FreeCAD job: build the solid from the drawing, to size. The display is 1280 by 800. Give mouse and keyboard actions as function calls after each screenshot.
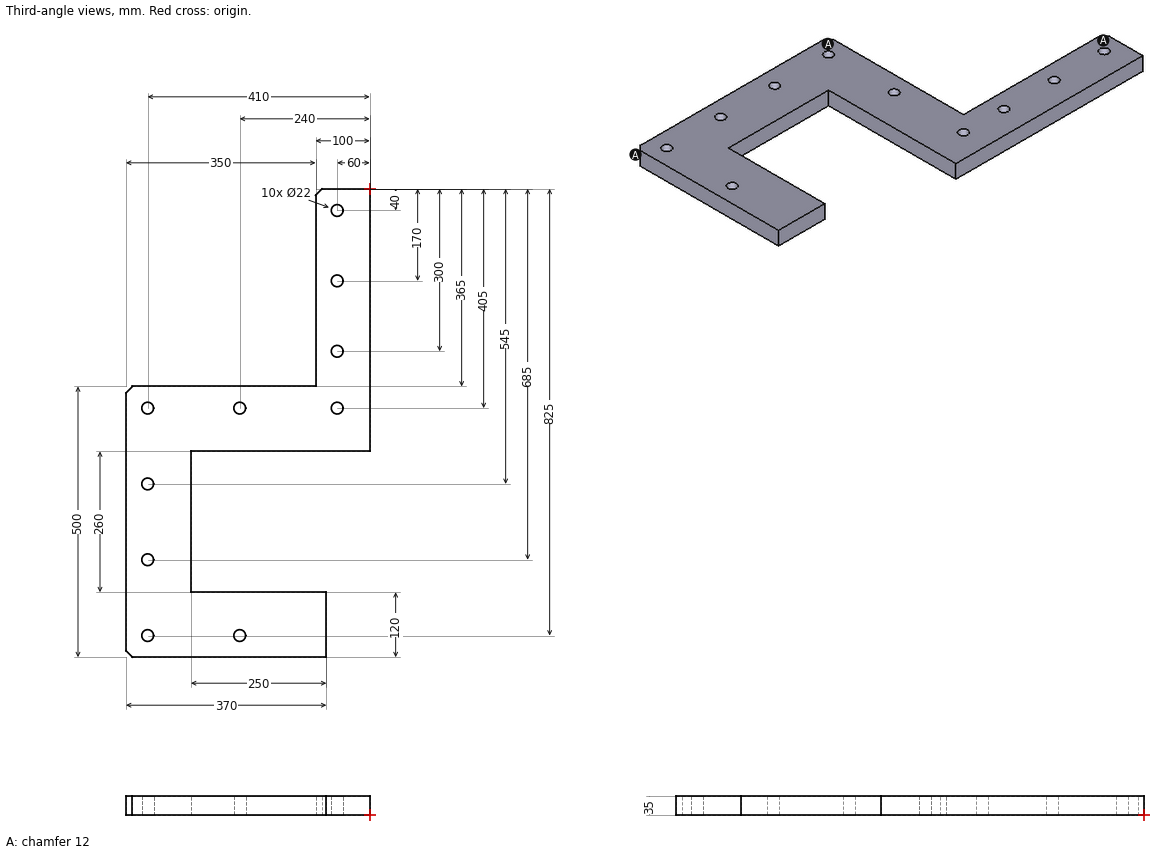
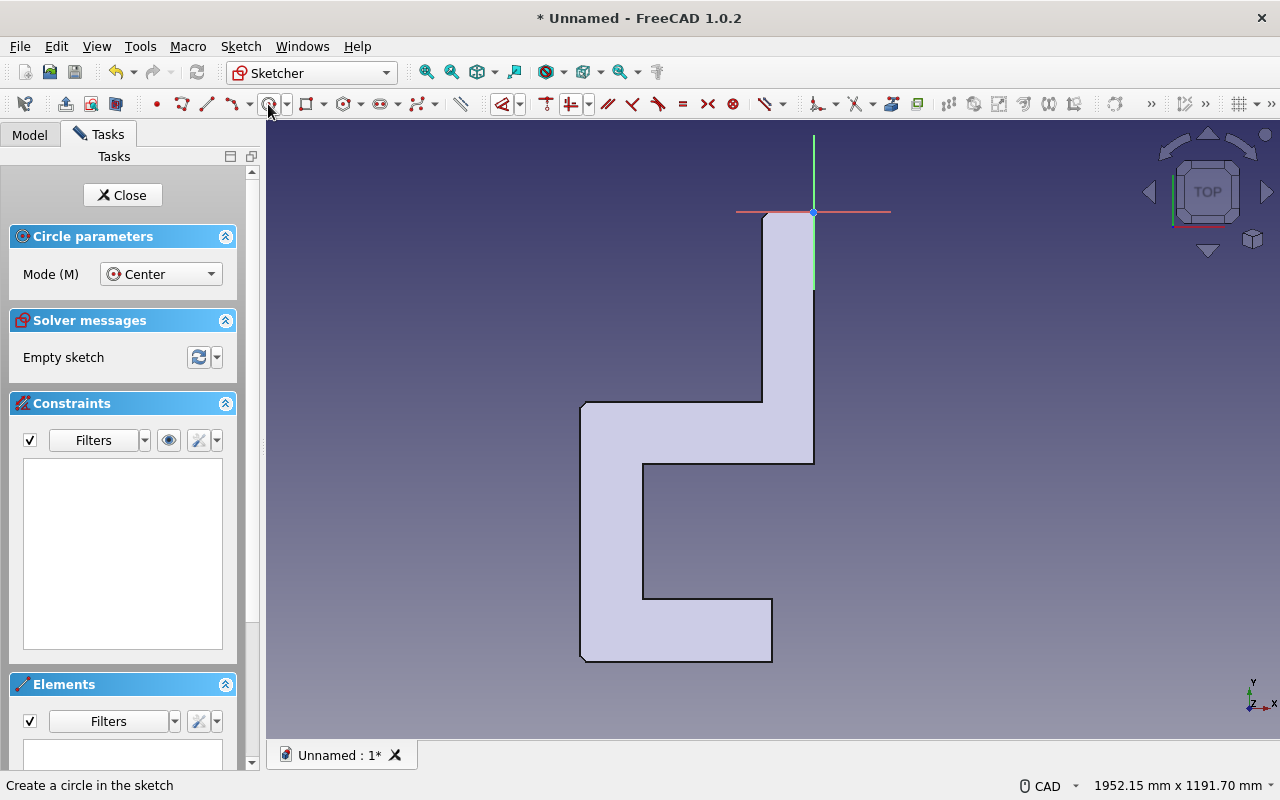
scroll(783, 233, up, 7)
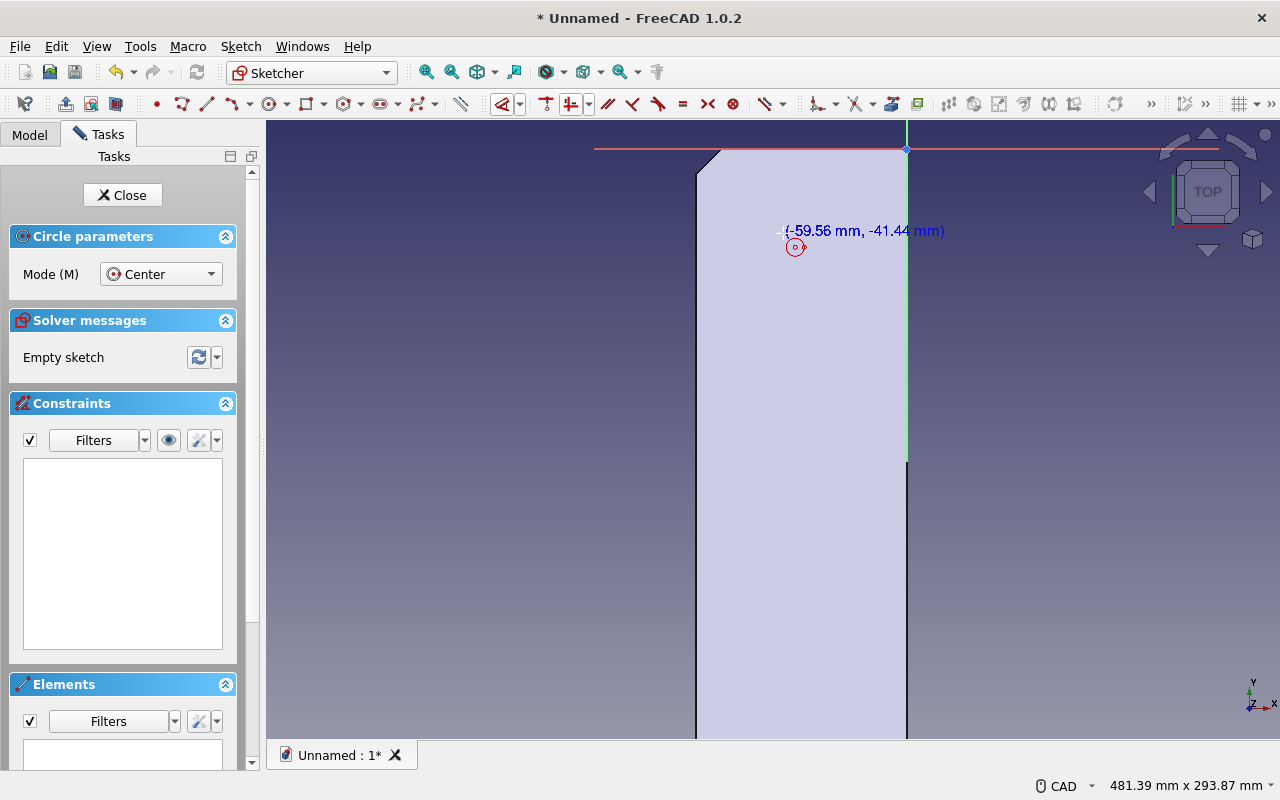
scroll(783, 233, down, 7)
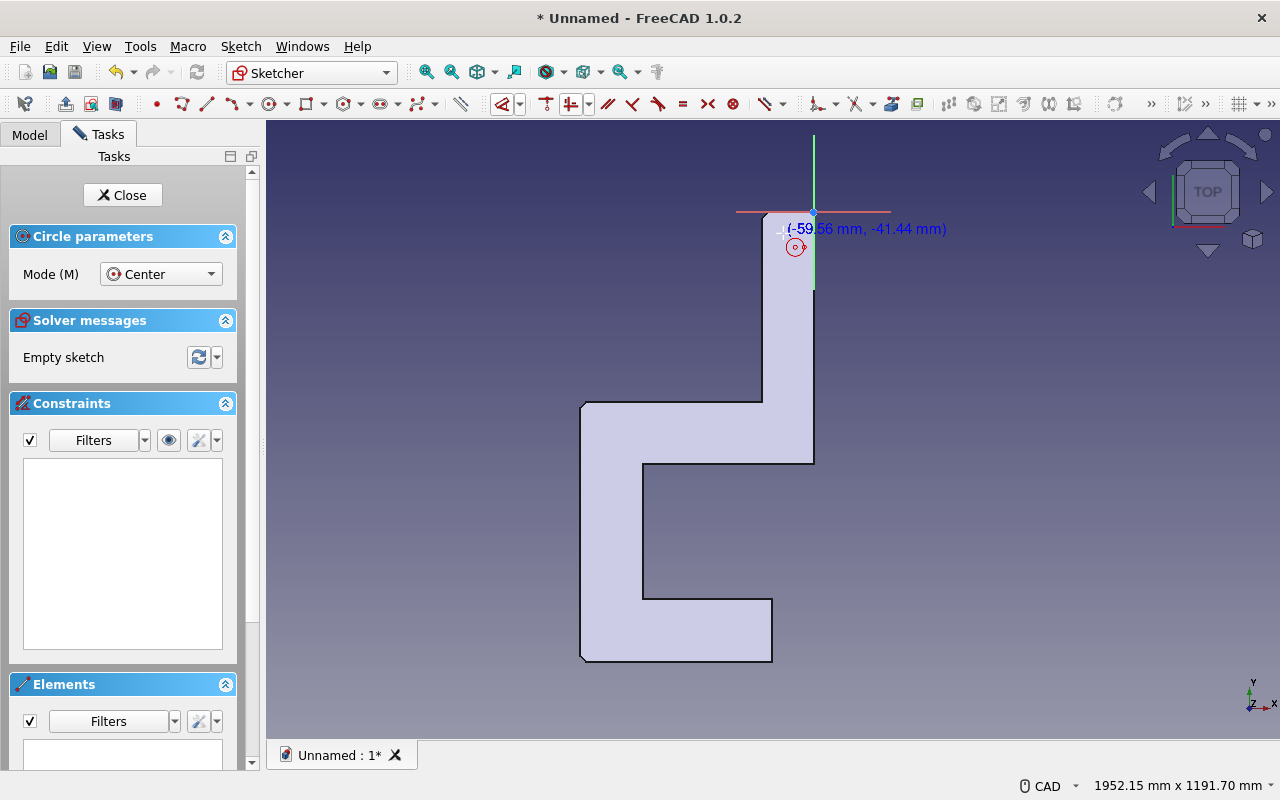
click(783, 233)
move(787, 229)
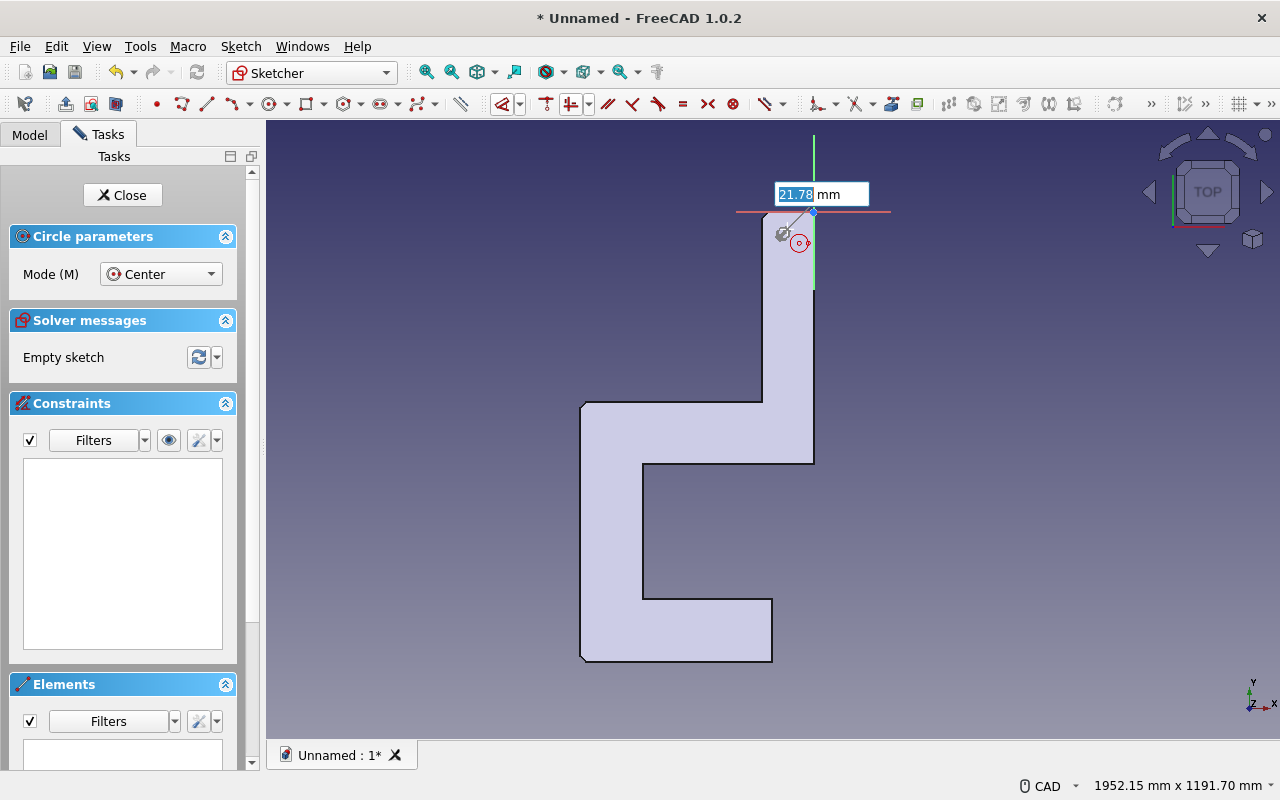
text(22)
key(Return)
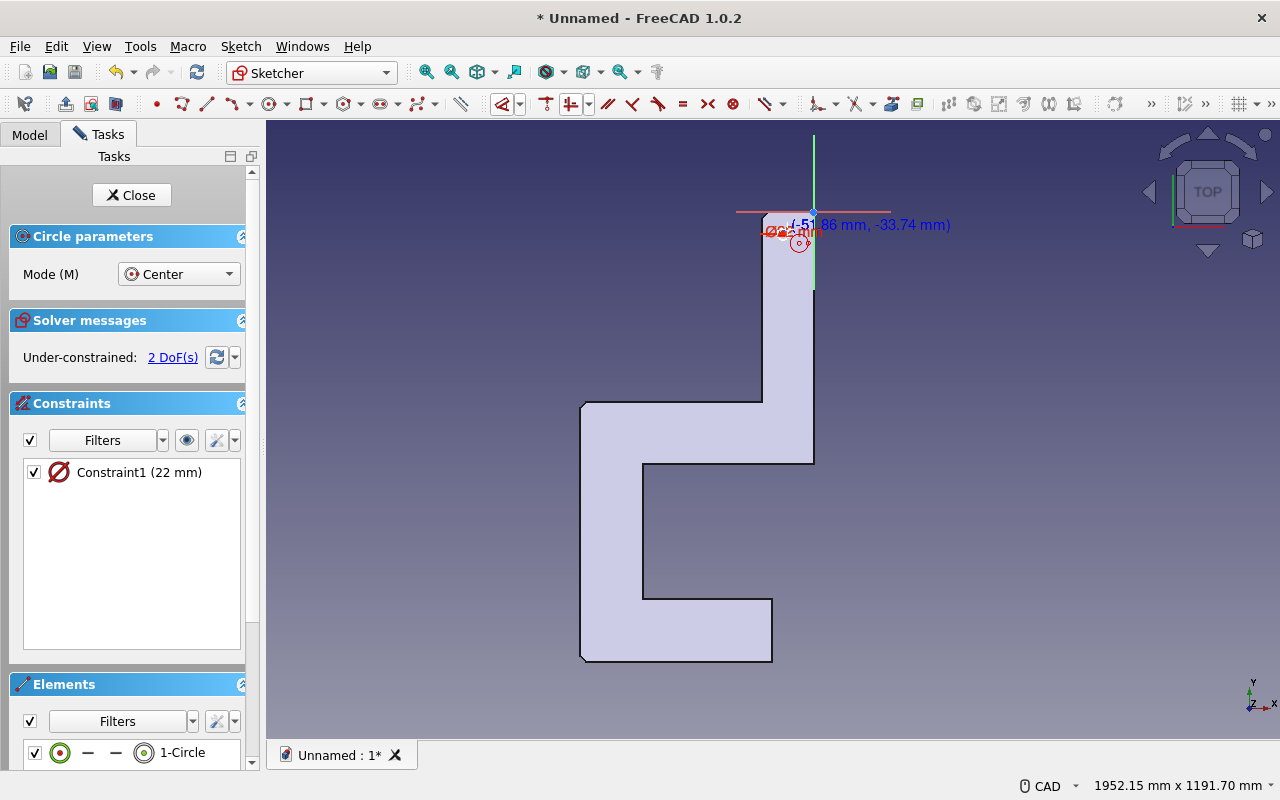
scroll(783, 301, up, 7)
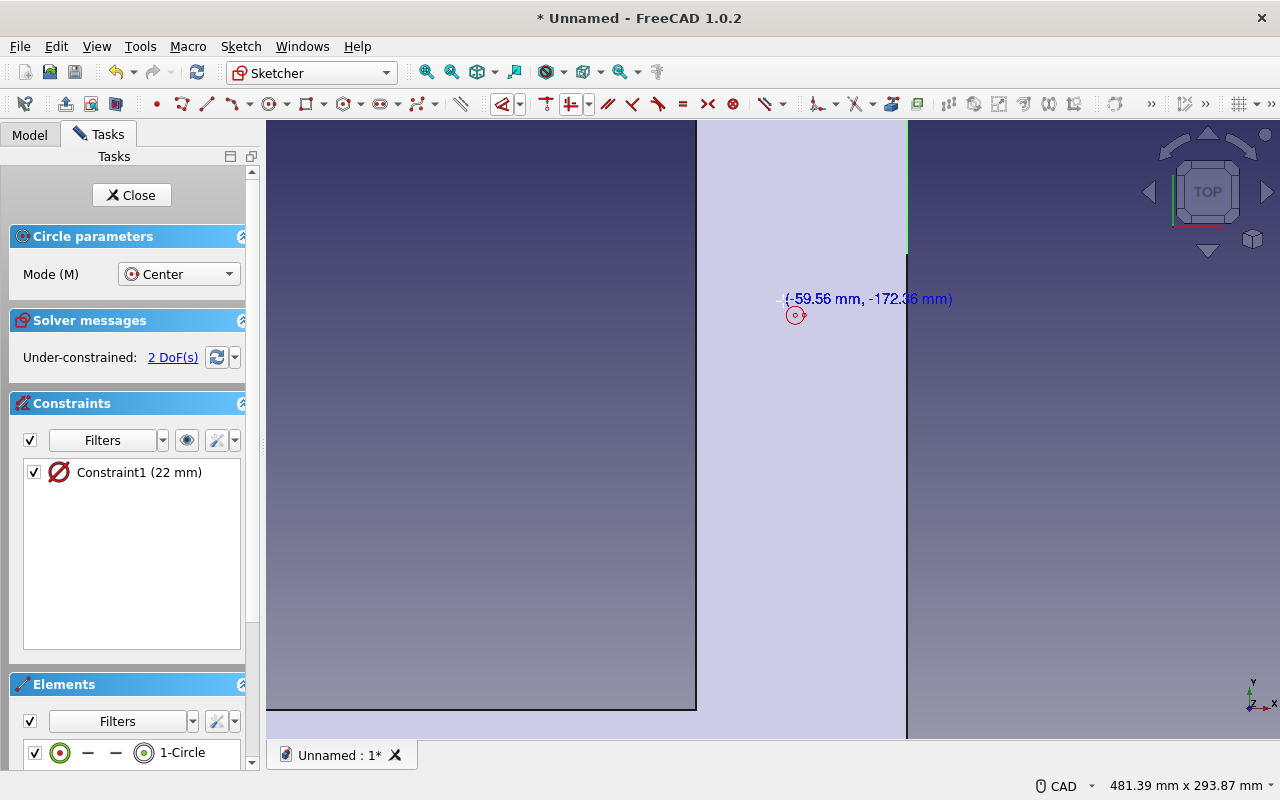
scroll(783, 301, down, 7)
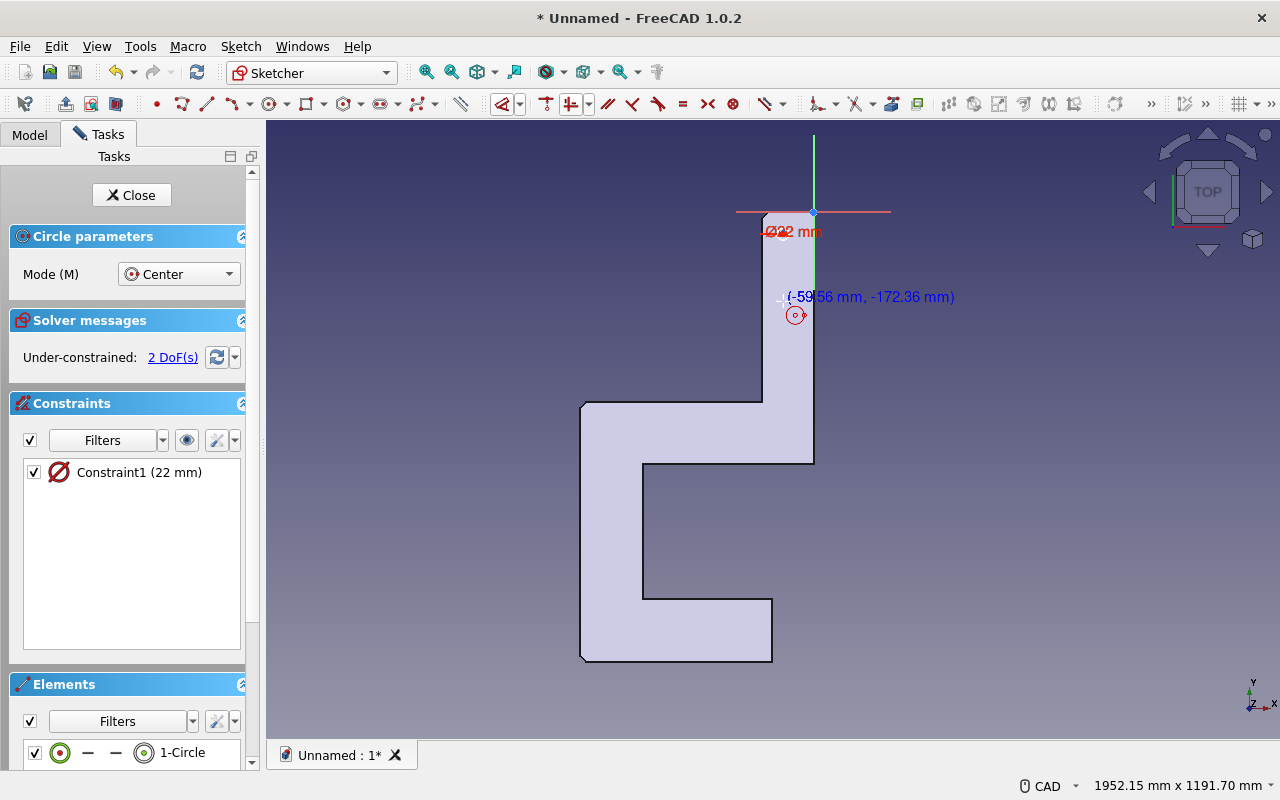
click(783, 301)
move(787, 297)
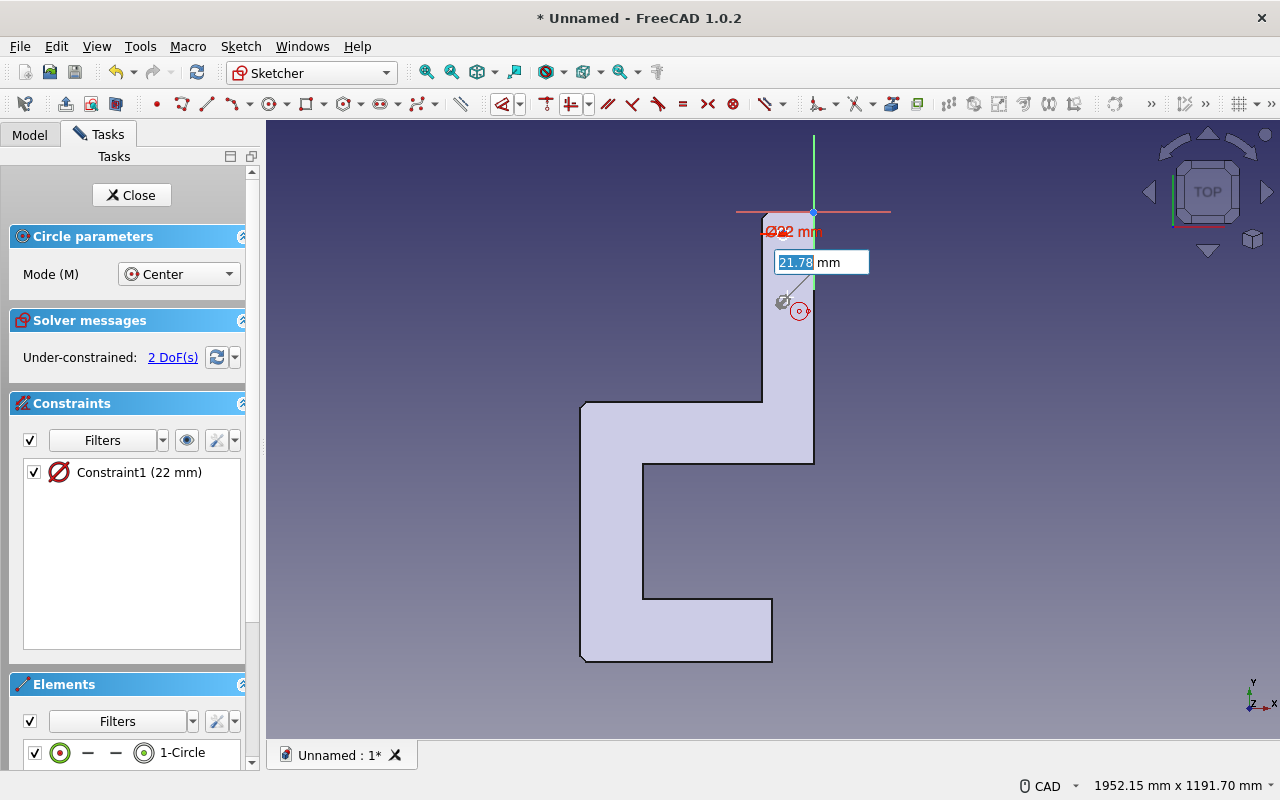
text(22)
key(Return)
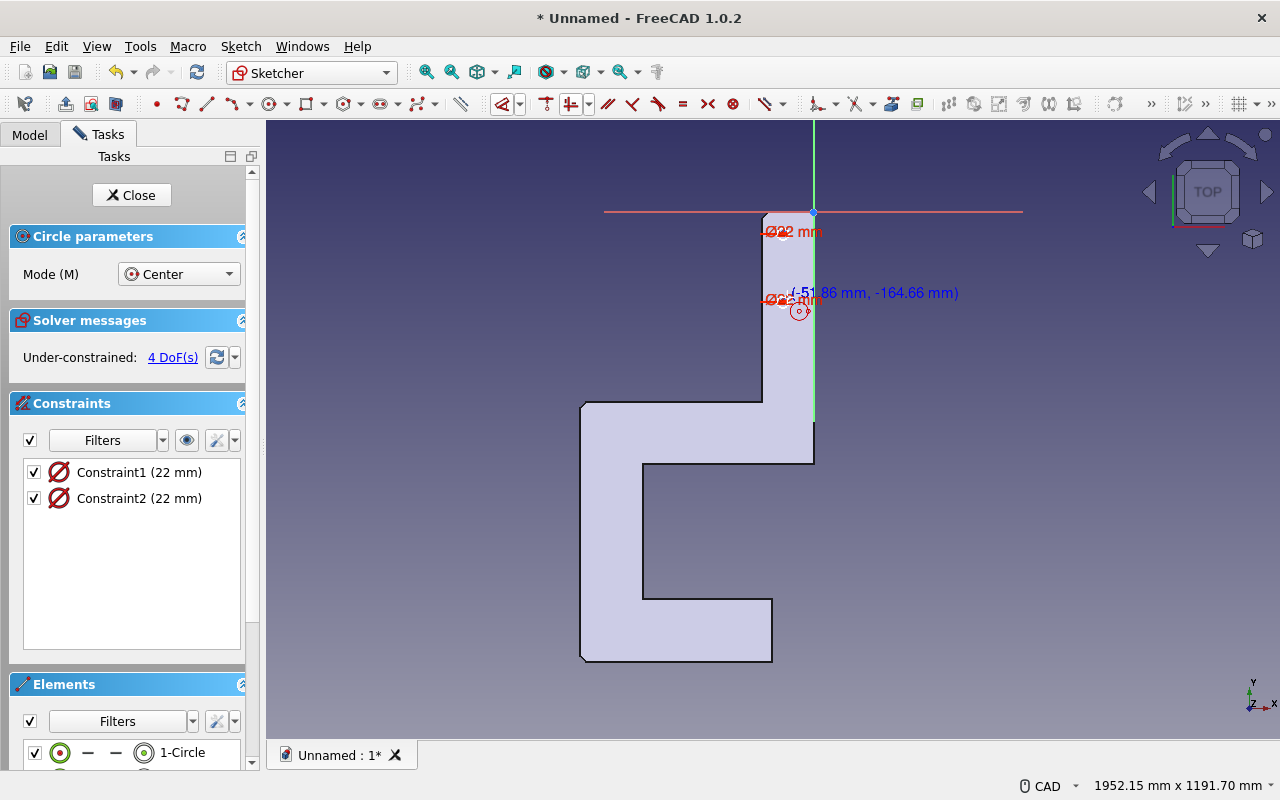
scroll(783, 368, up, 7)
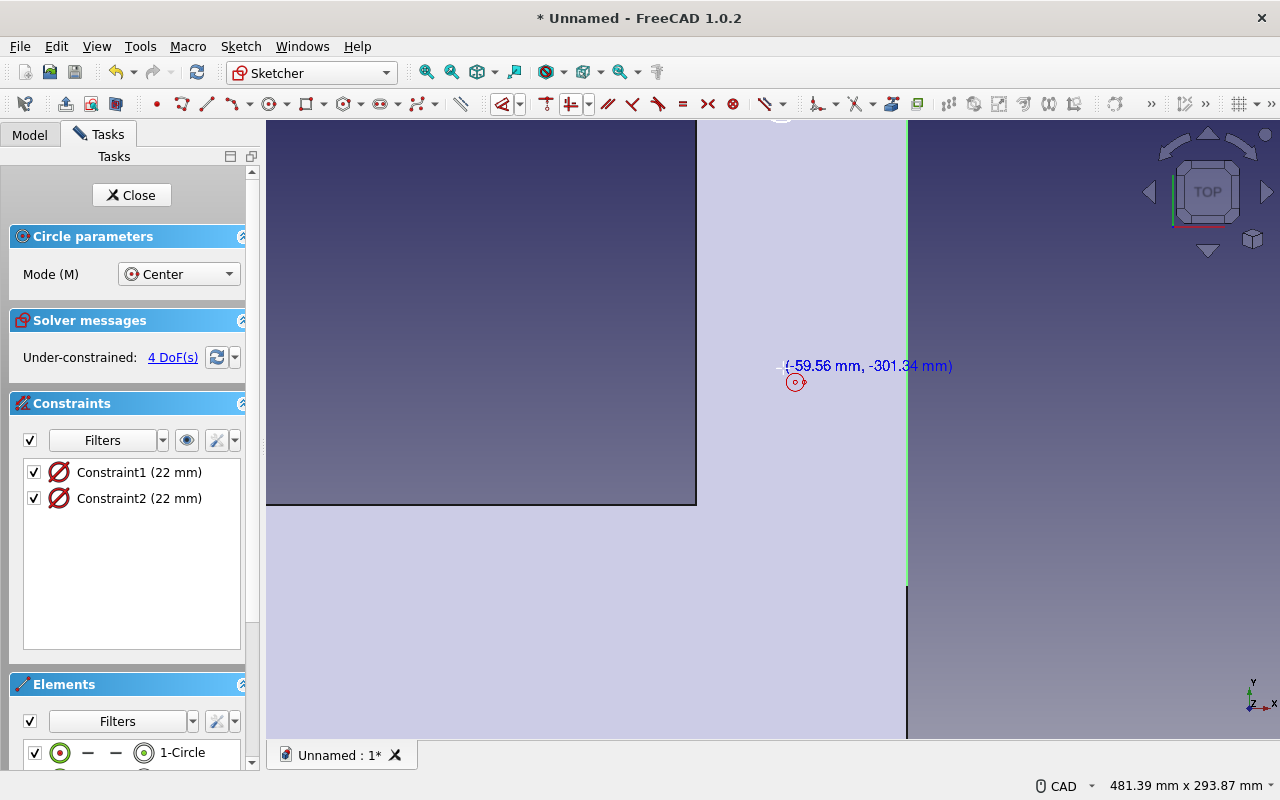
scroll(783, 368, down, 7)